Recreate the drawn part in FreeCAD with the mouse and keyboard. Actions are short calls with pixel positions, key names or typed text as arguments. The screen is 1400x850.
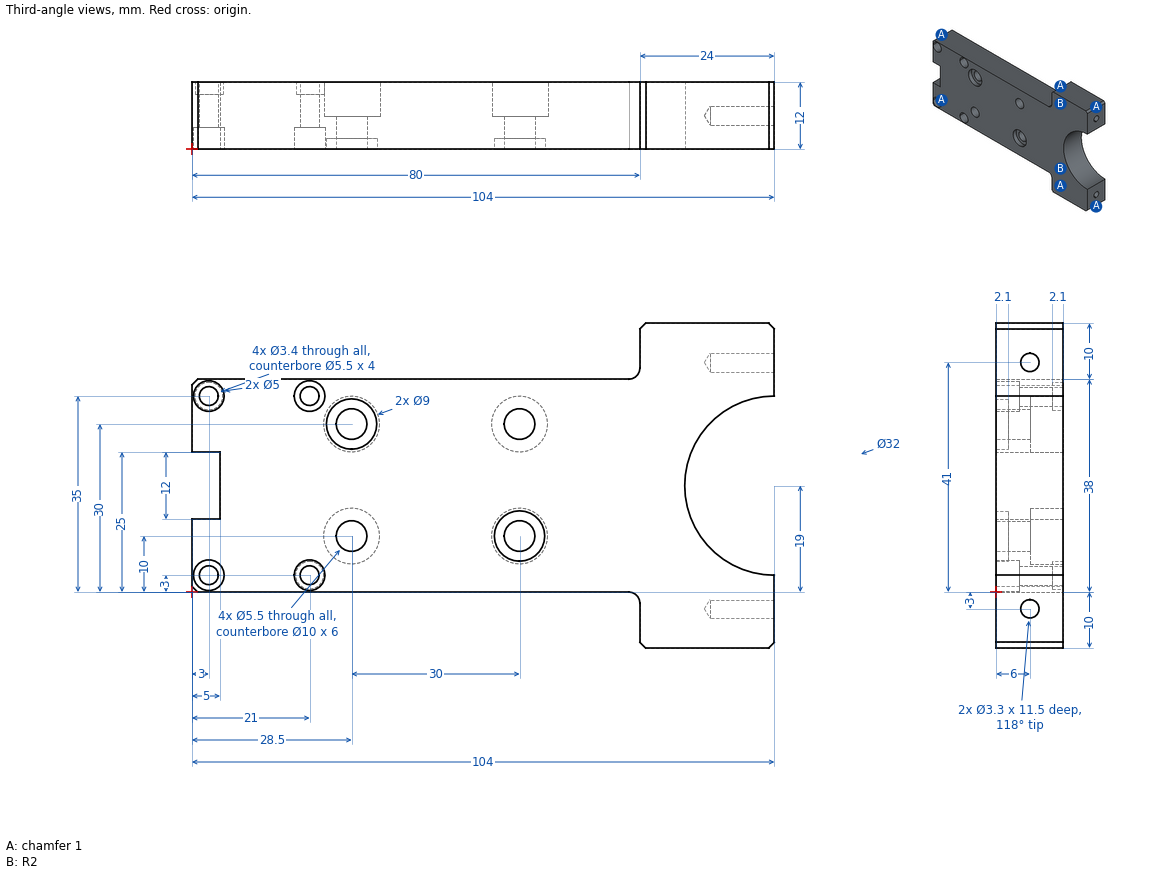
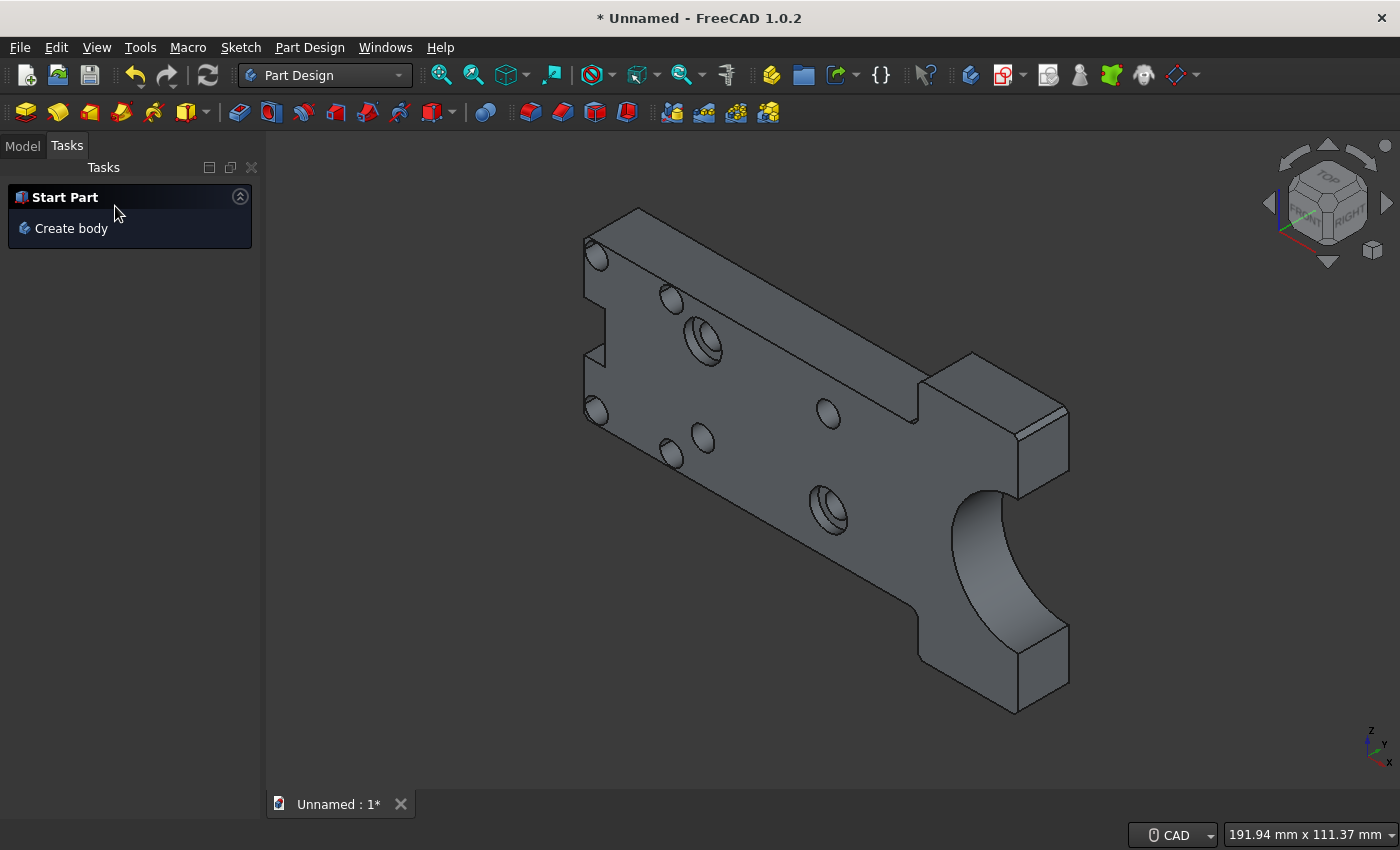
click(1043, 667)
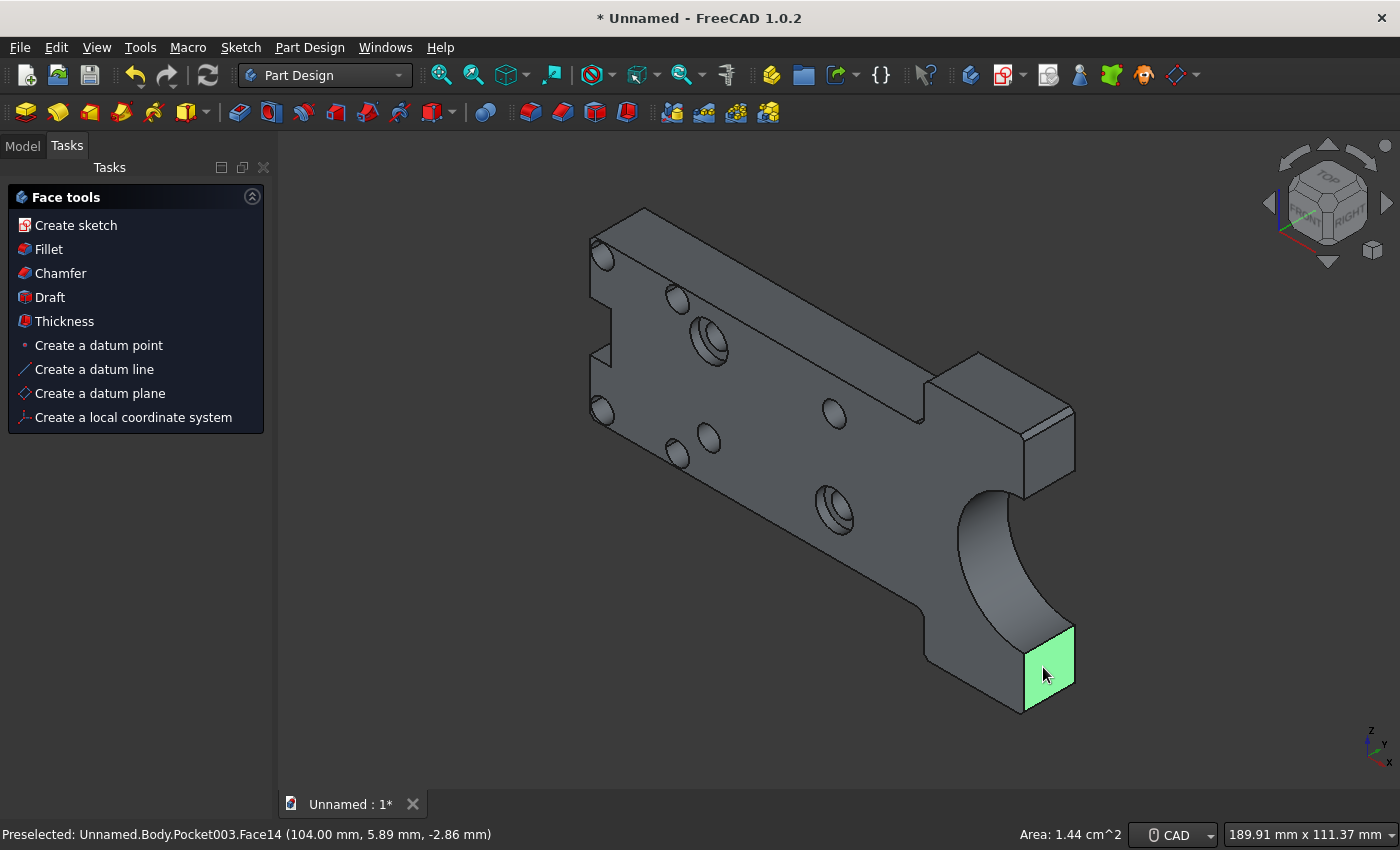
click(1004, 76)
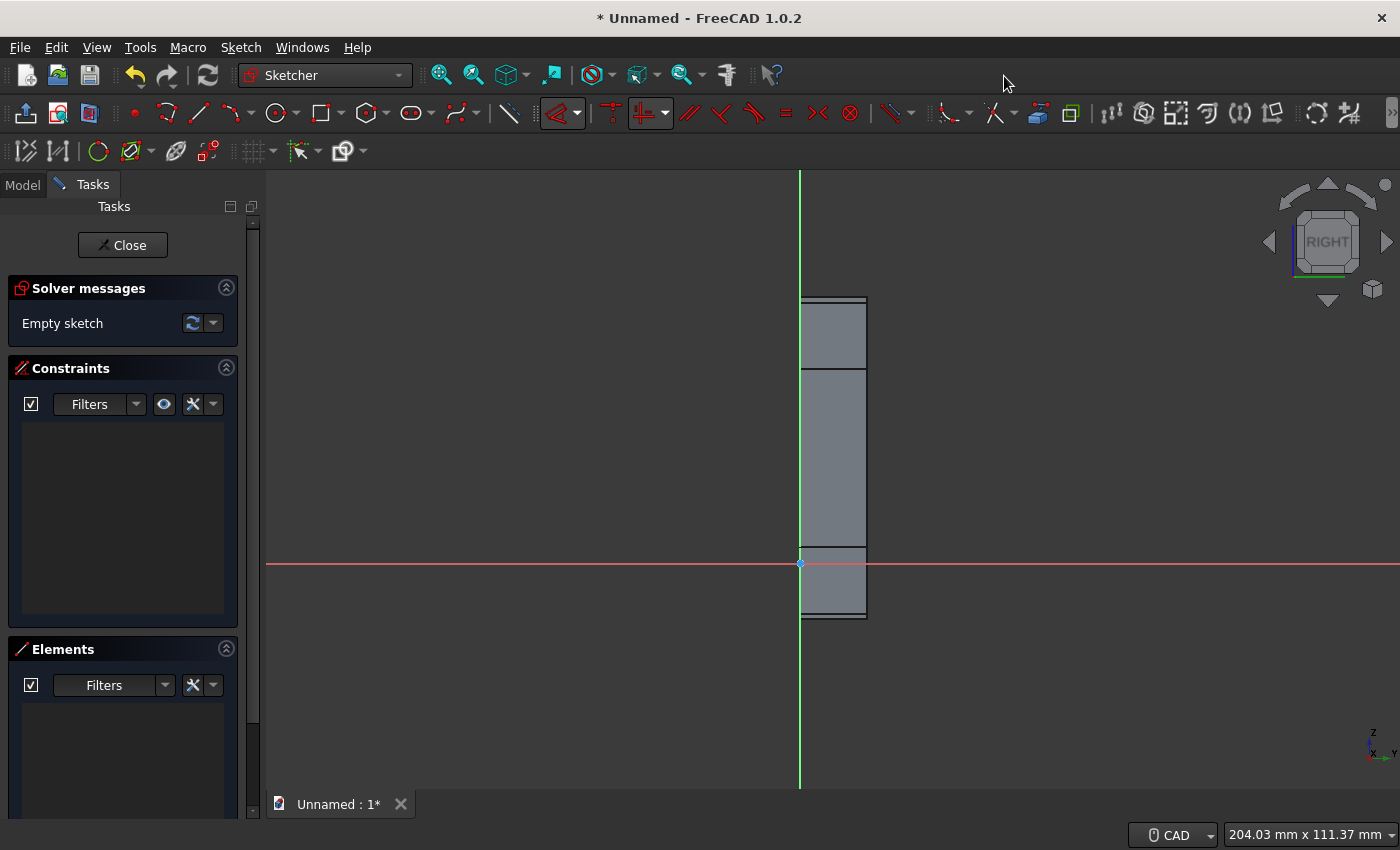
scroll(938, 415, up, 2)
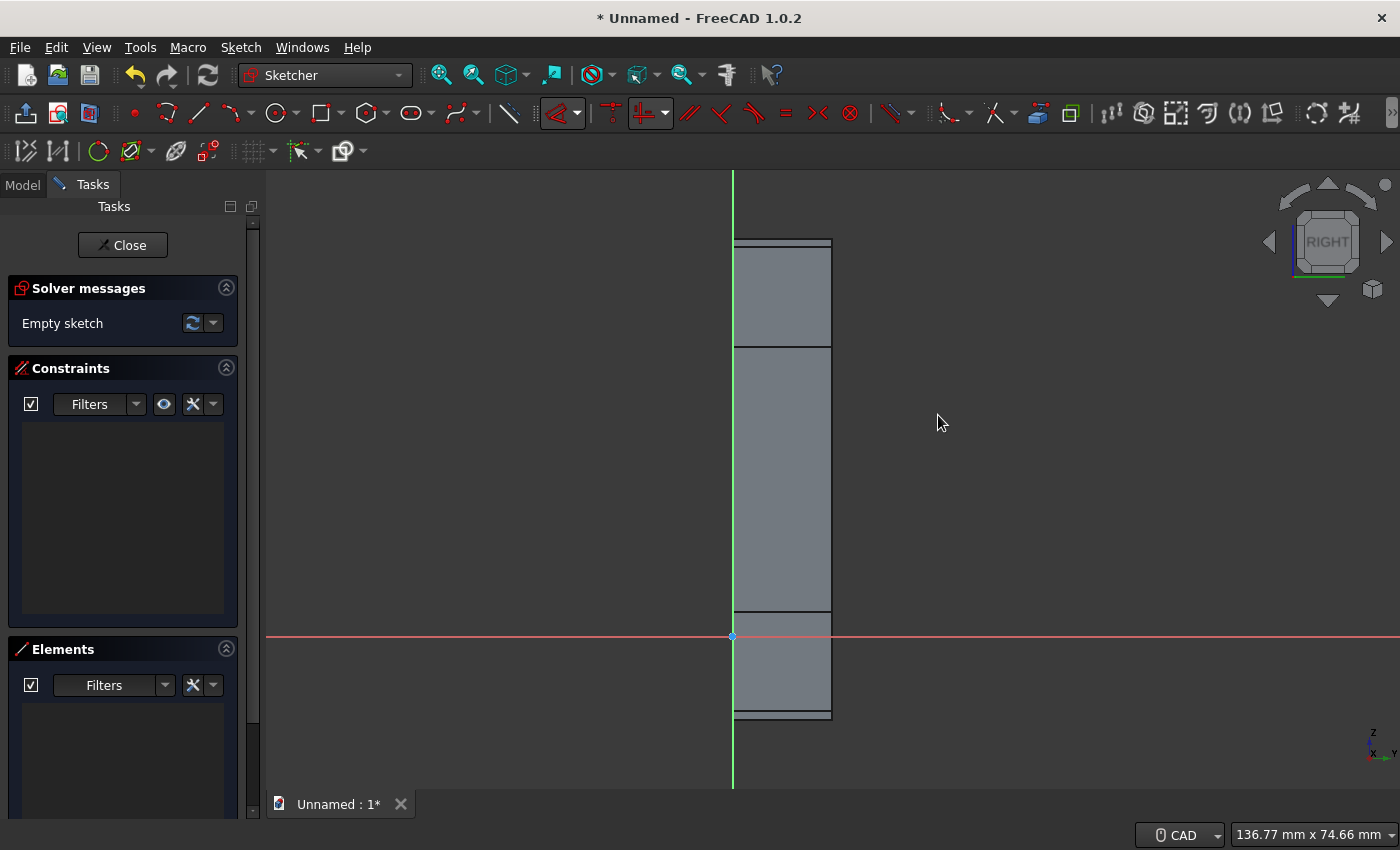
click(276, 114)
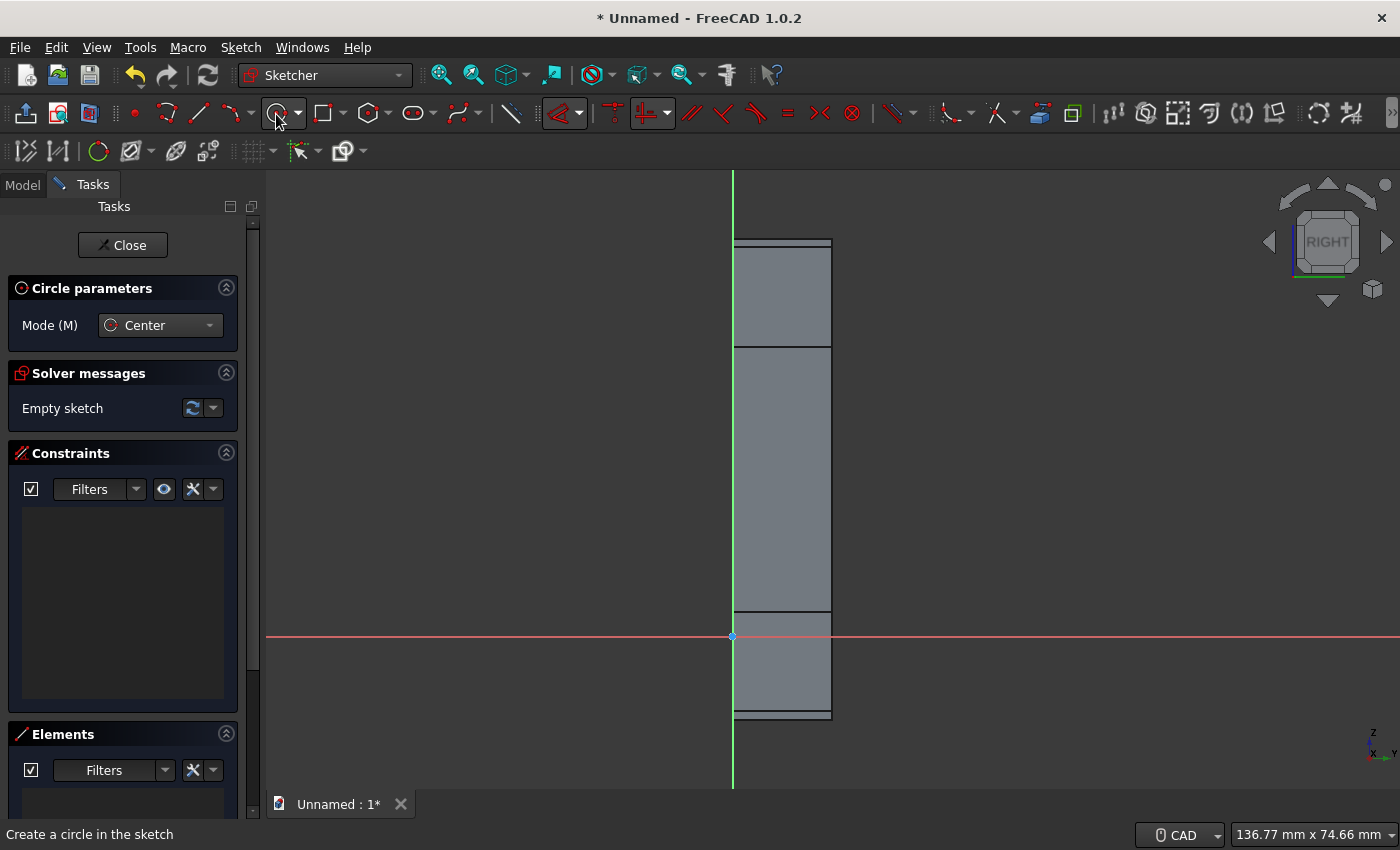
scroll(782, 662, up, 3)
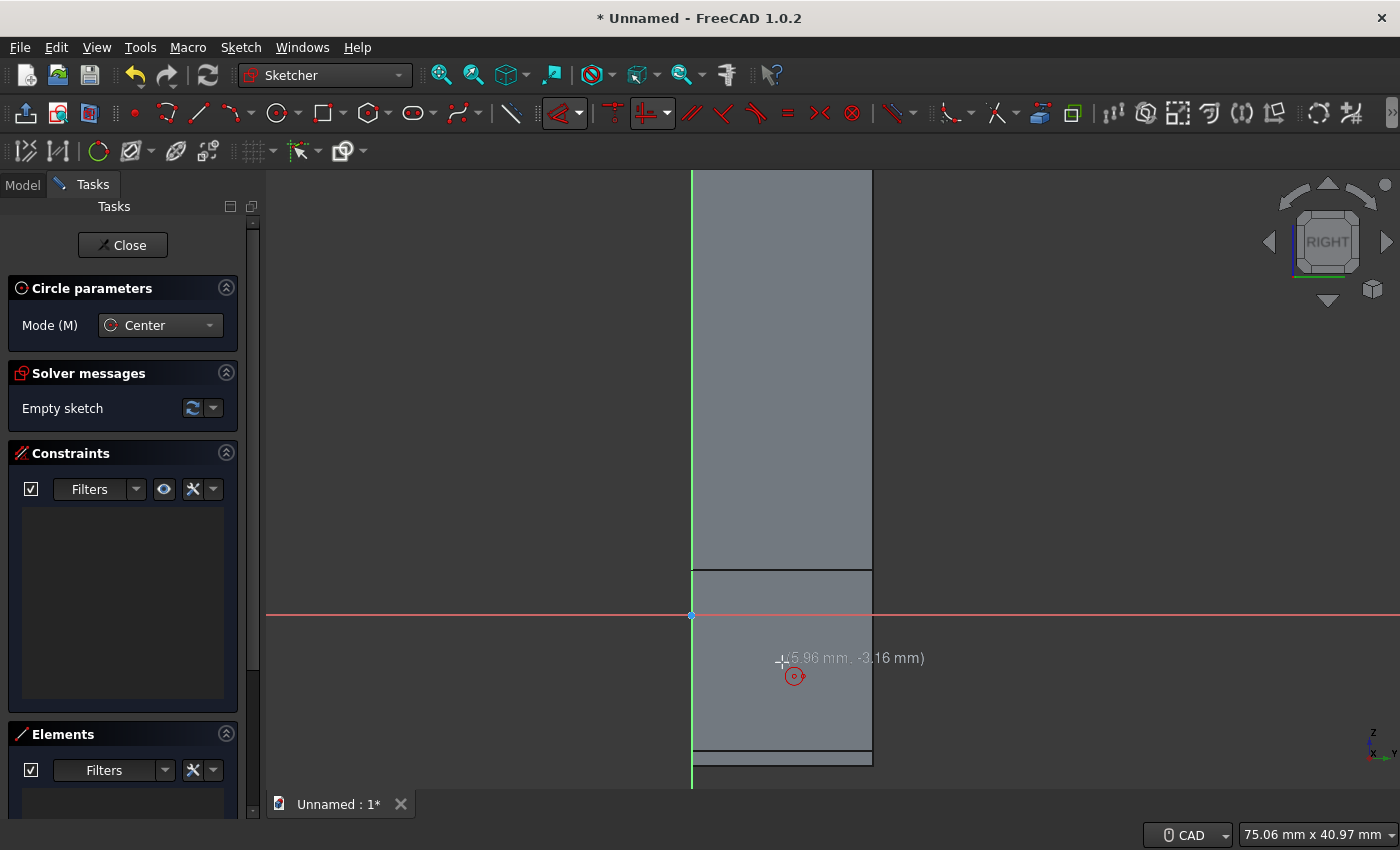
click(782, 661)
click(800, 643)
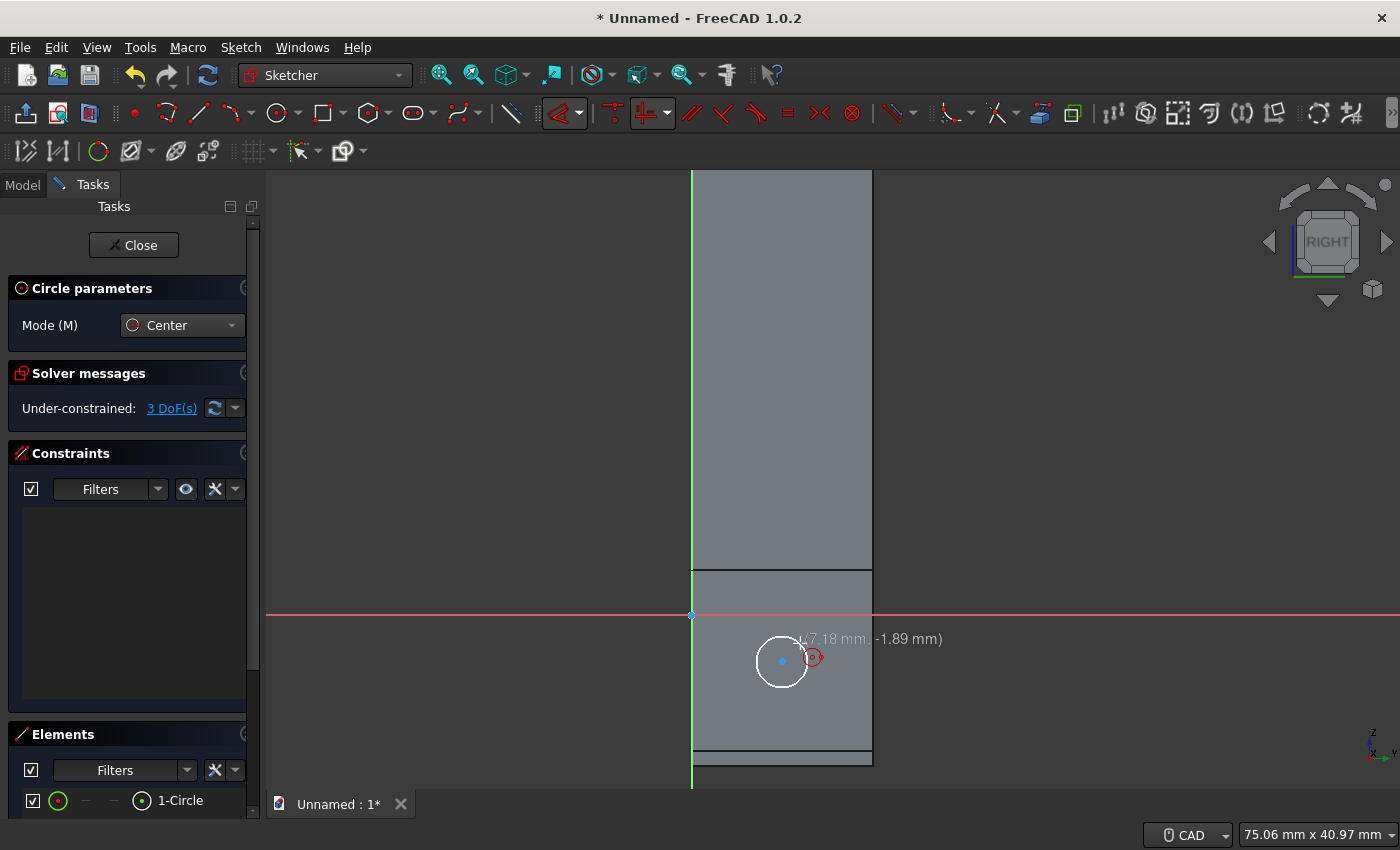
scroll(783, 663, down, 3)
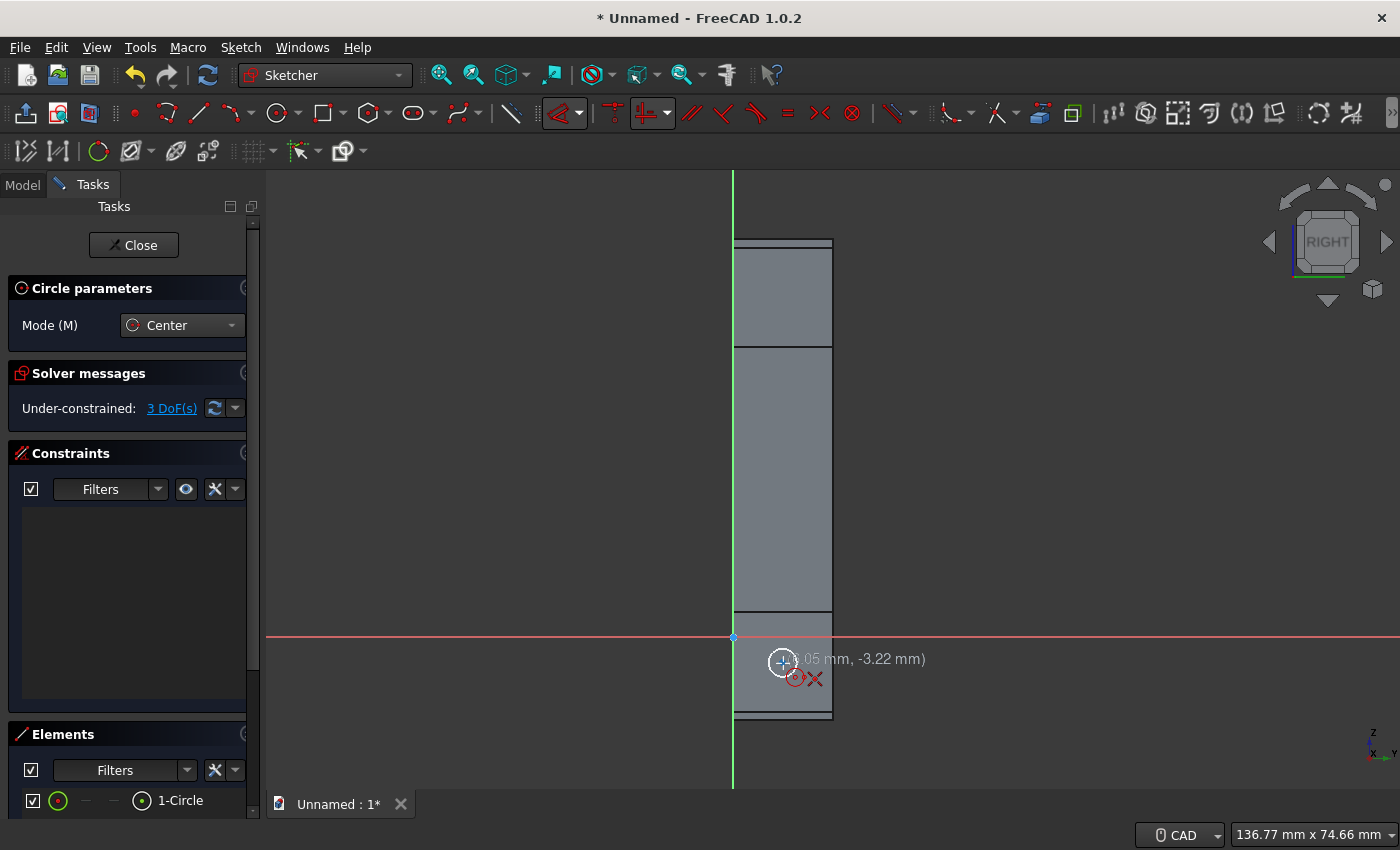
scroll(783, 297, up, 3)